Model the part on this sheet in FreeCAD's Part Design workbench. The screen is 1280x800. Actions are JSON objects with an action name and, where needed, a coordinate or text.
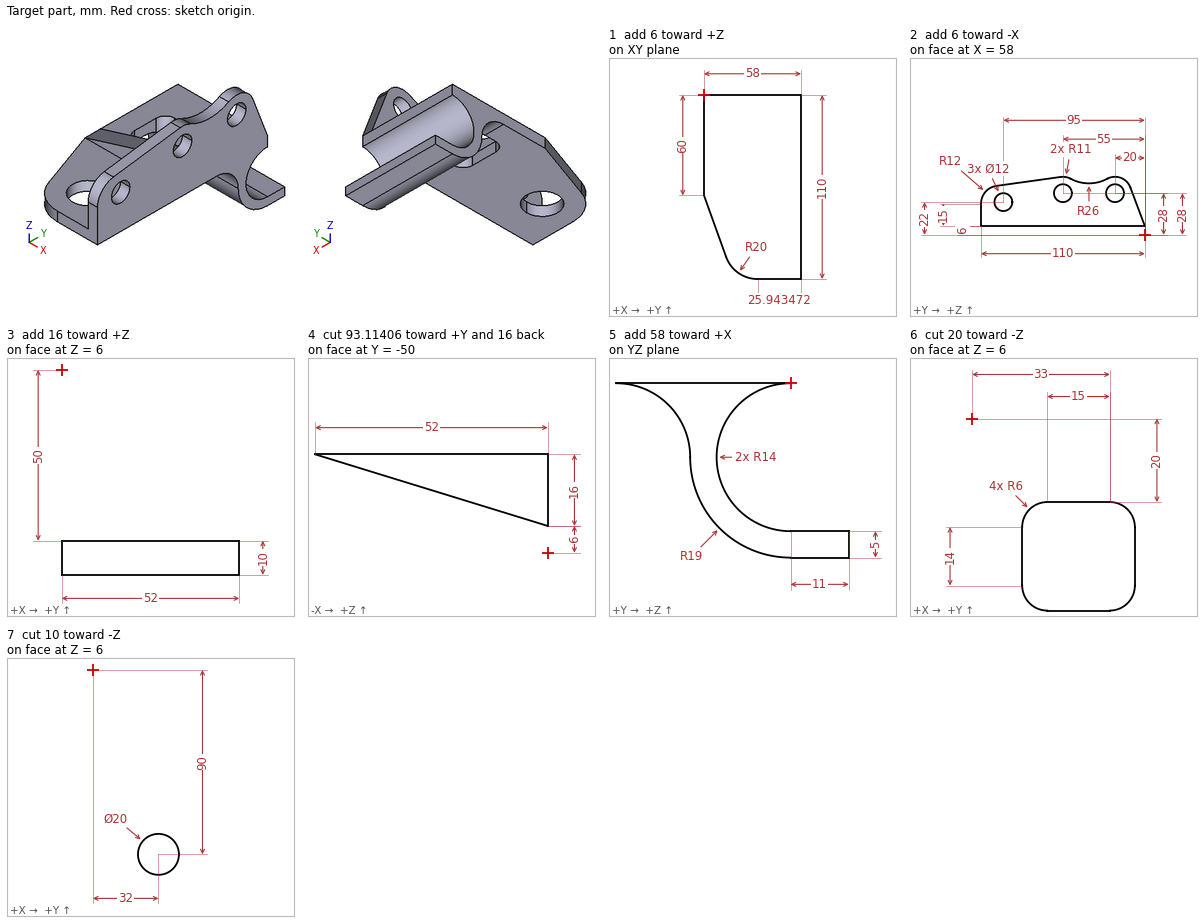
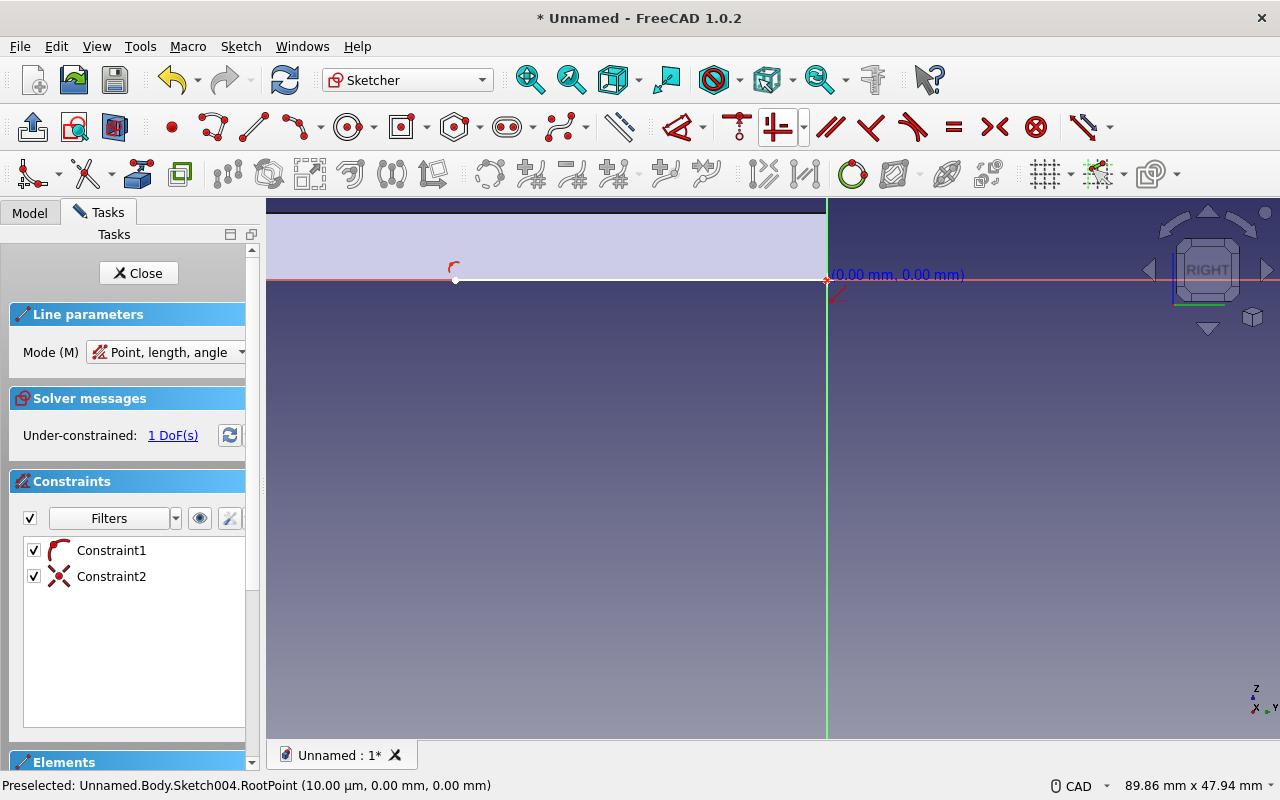
{"action": "left_click", "coordinate": [213, 128]}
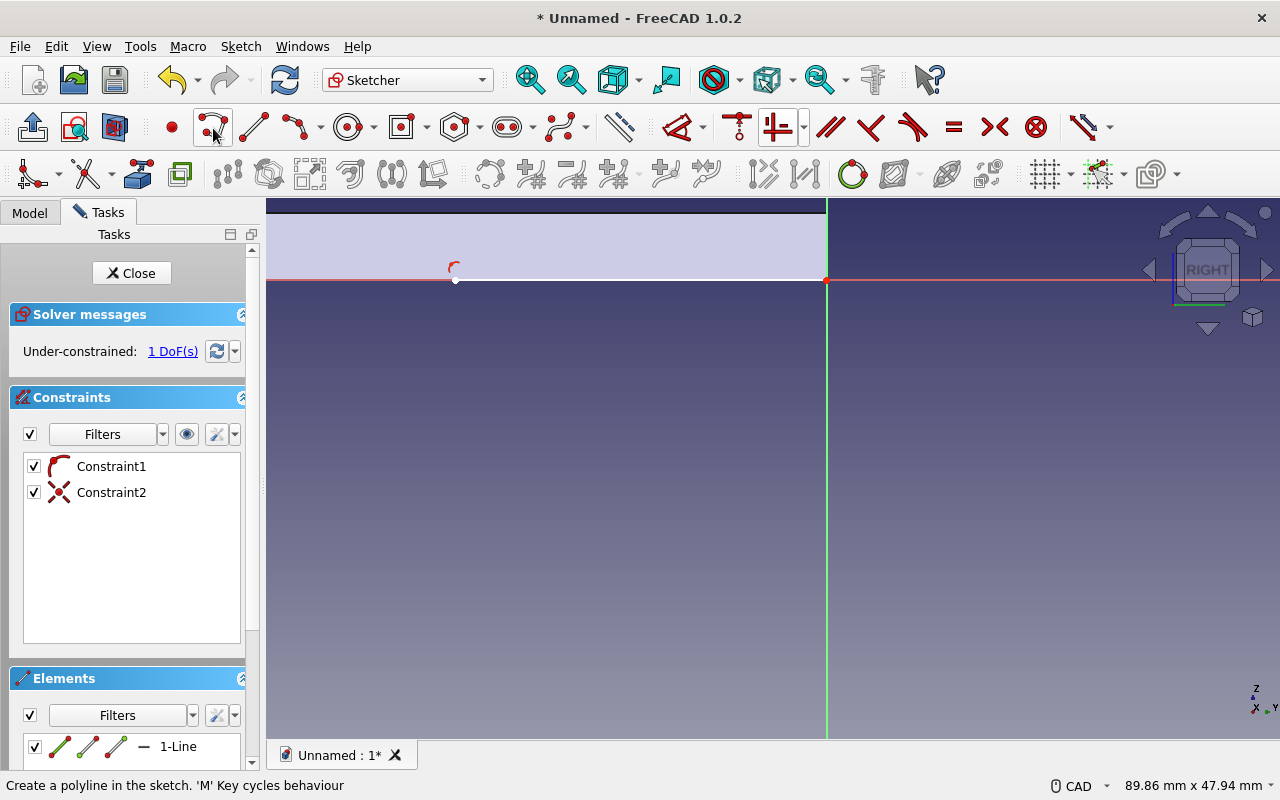
{"action": "left_click", "coordinate": [827, 596]}
{"action": "left_click", "coordinate": [951, 596]}
{"action": "left_click", "coordinate": [951, 653]}
{"action": "left_click", "coordinate": [827, 653]}
{"action": "right_click", "coordinate": [827, 653]}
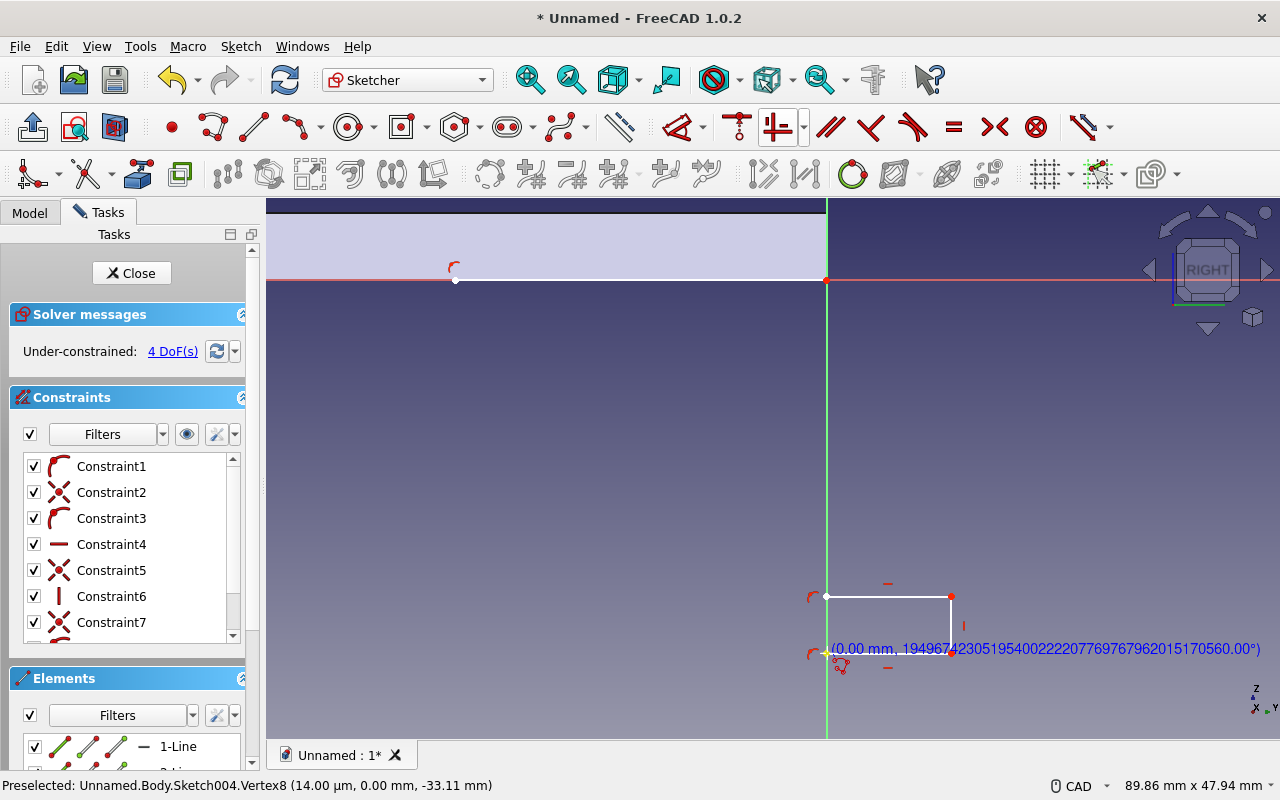
{"action": "left_click", "coordinate": [294, 128]}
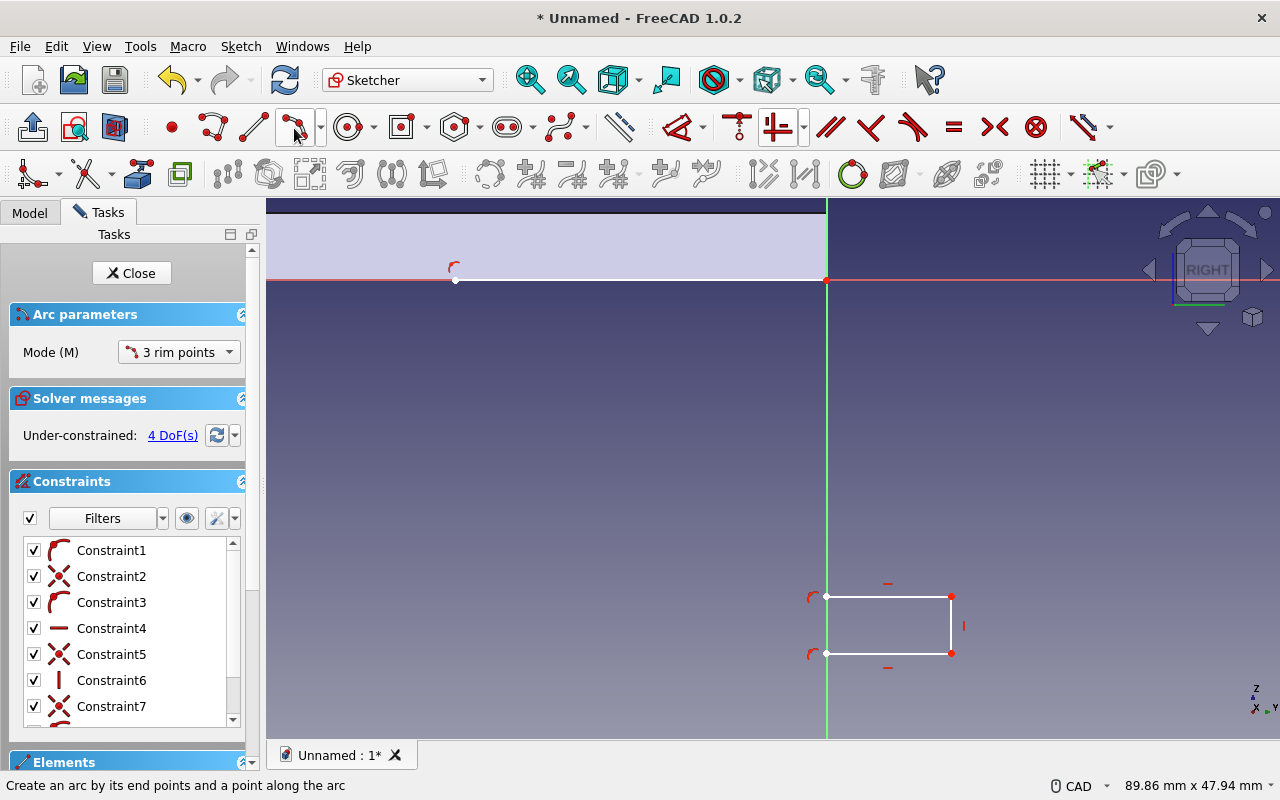
{"action": "left_click", "coordinate": [827, 280]}
{"action": "left_click", "coordinate": [827, 597]}
{"action": "left_click", "coordinate": [669, 438]}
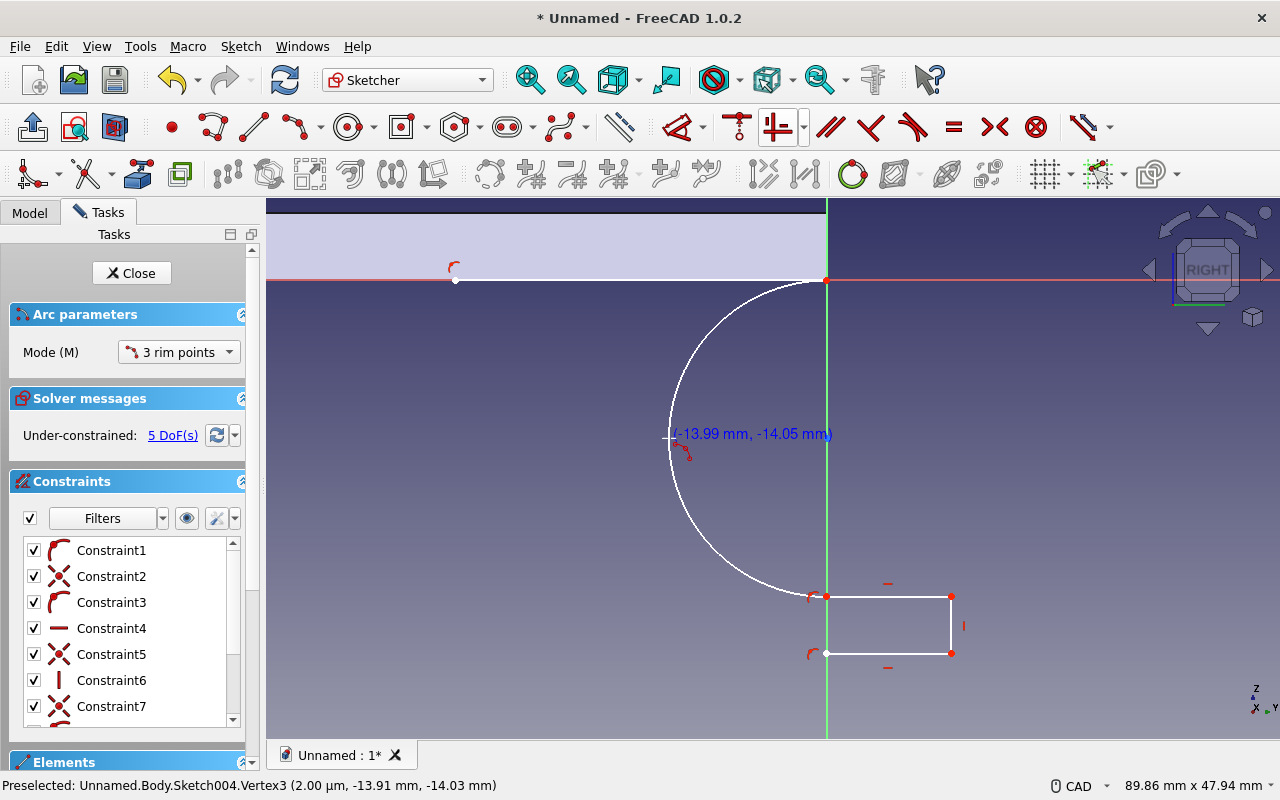
{"action": "left_click", "coordinate": [827, 654]}
{"action": "left_click", "coordinate": [613, 438]}
{"action": "left_click", "coordinate": [675, 590]}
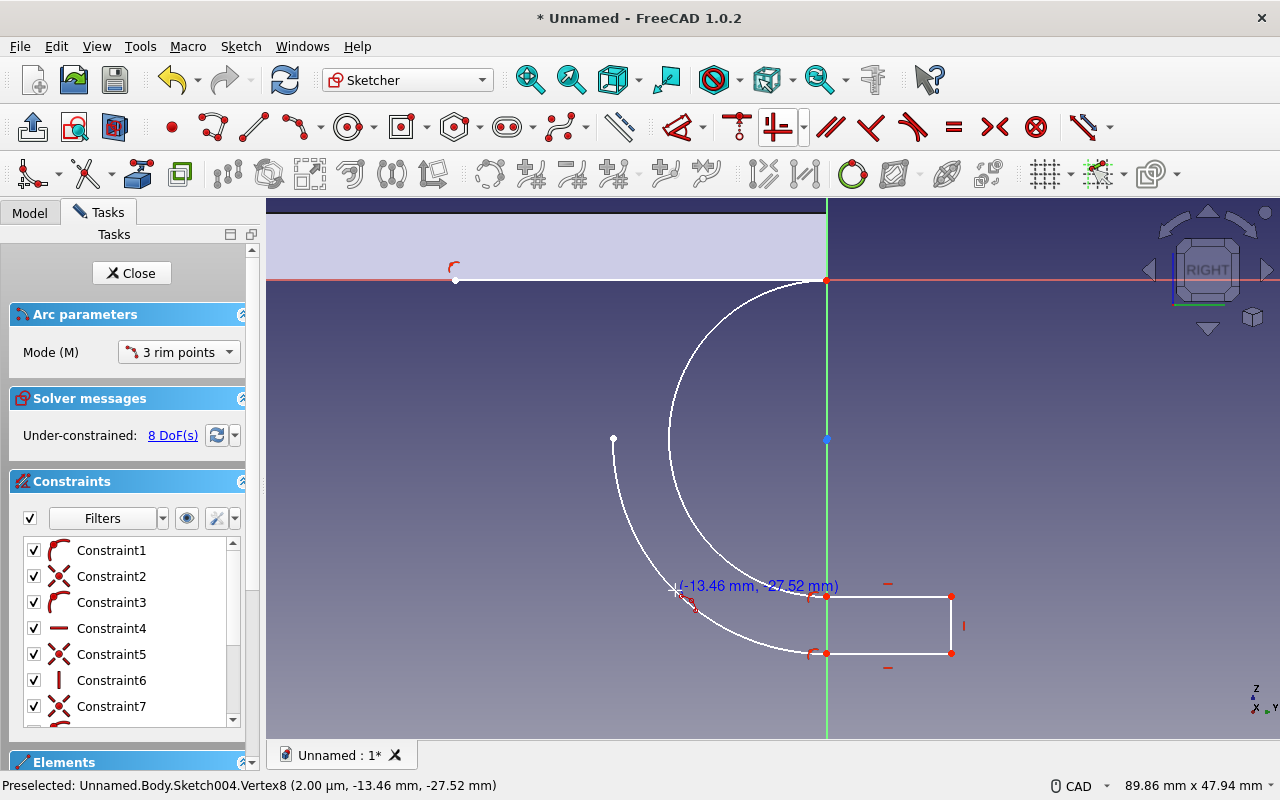
{"action": "left_click", "coordinate": [613, 439]}
{"action": "left_click", "coordinate": [455, 280]}
{"action": "left_click", "coordinate": [566, 327]}
{"action": "key", "text": "Escape"}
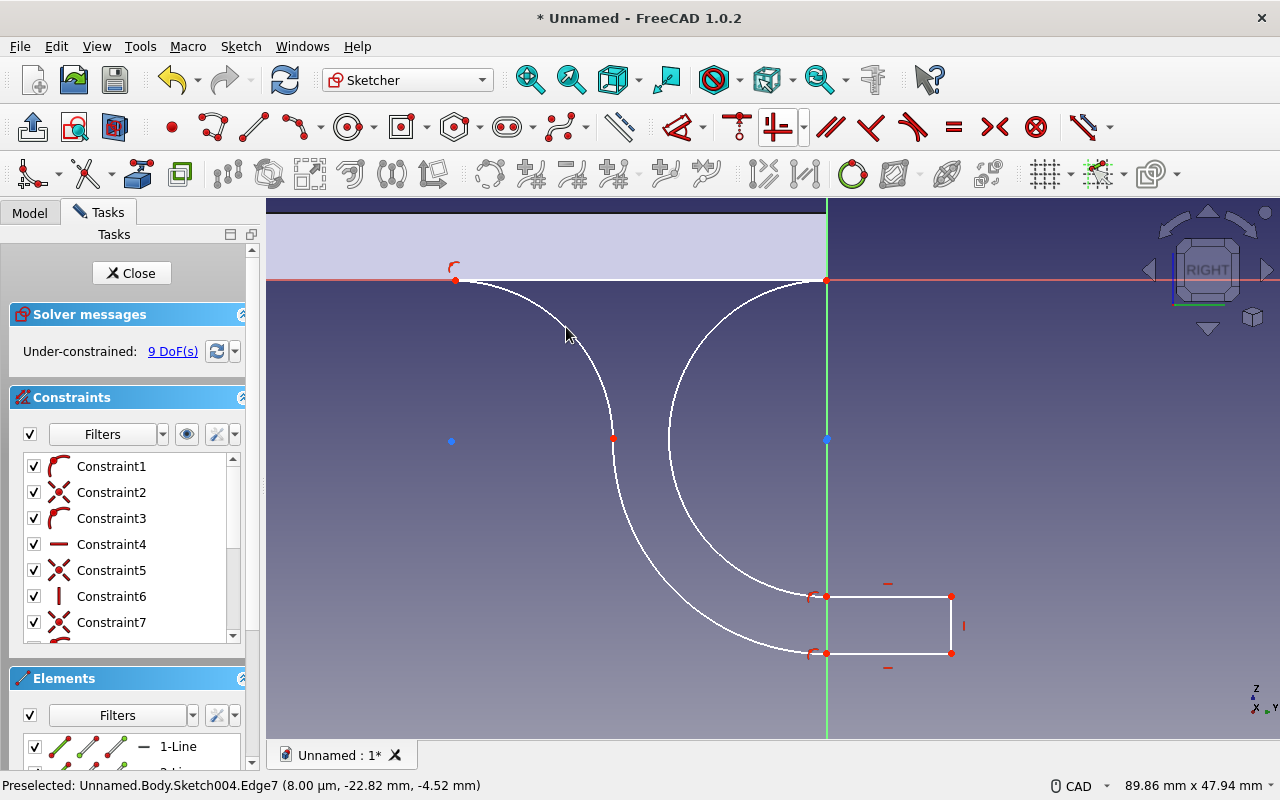
{"action": "left_click", "coordinate": [567, 280]}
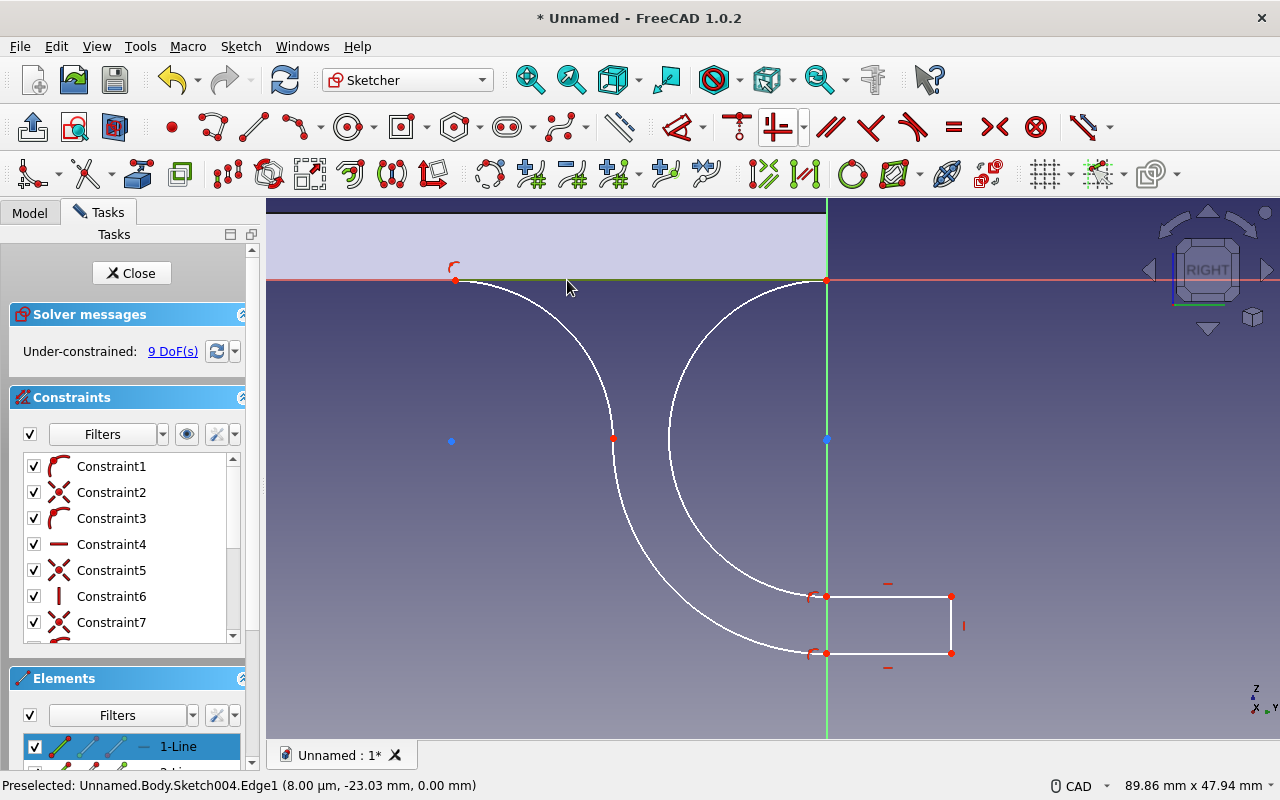
{"action": "left_click", "coordinate": [699, 346]}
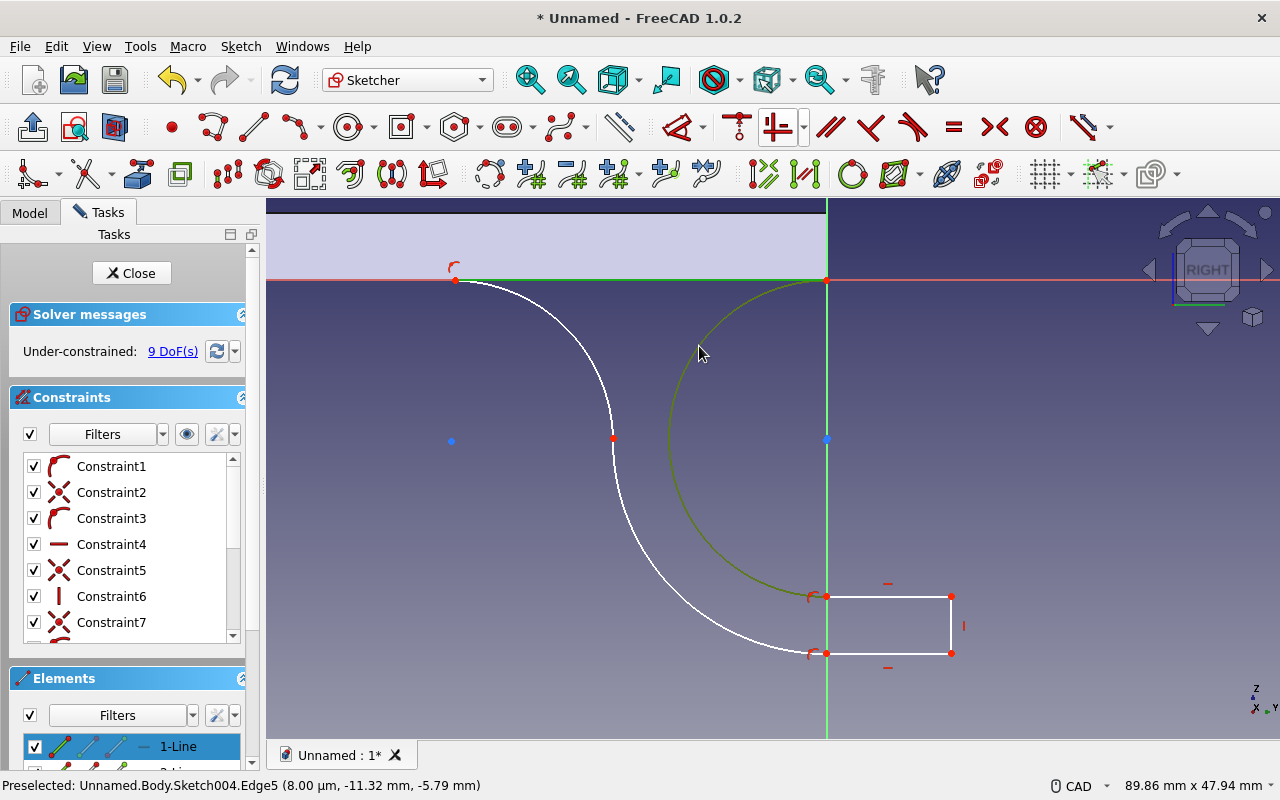
{"action": "left_click", "coordinate": [913, 128]}